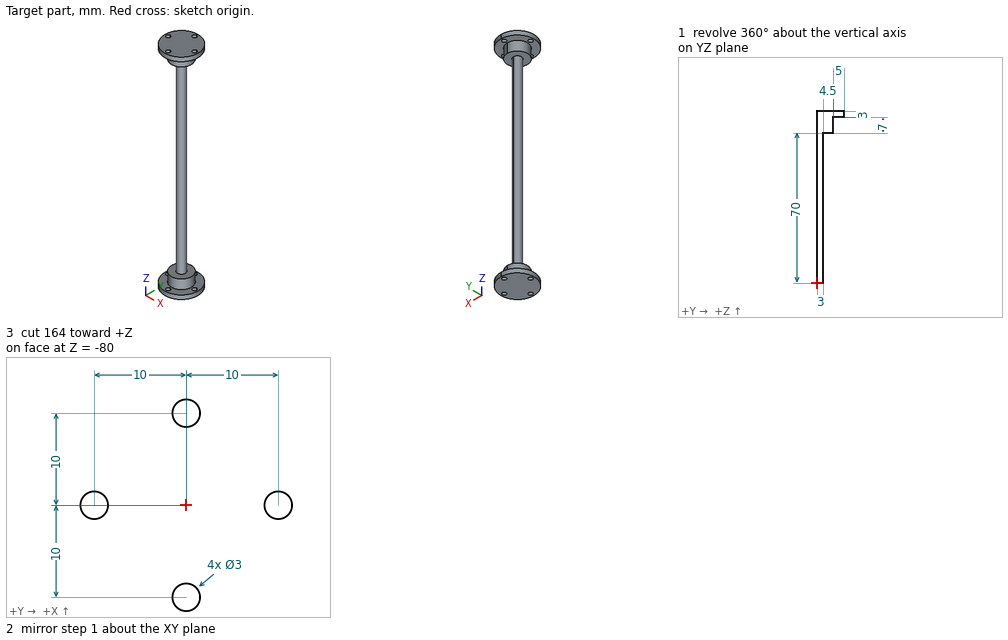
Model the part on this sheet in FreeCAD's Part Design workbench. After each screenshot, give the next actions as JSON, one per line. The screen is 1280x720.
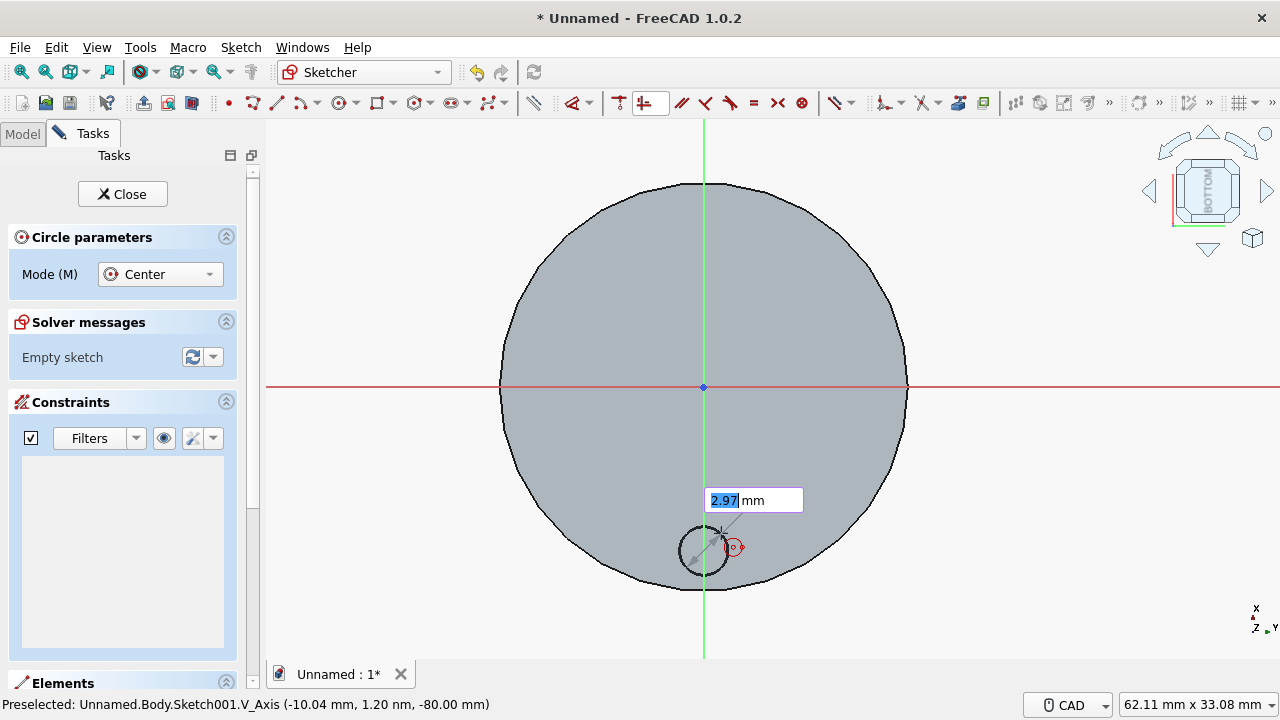
{"action": "type", "text": "3"}
{"action": "key", "text": "Return"}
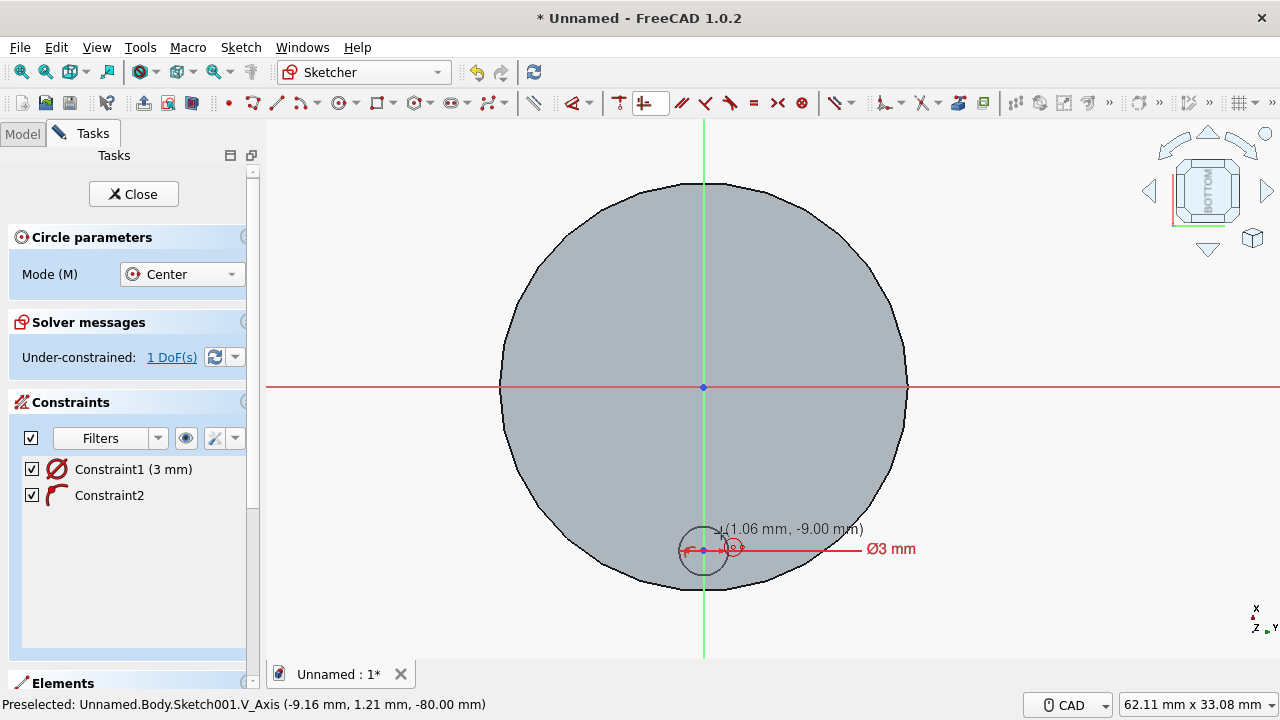
{"action": "left_click", "coordinate": [541, 387]}
{"action": "mouse_move", "coordinate": [558, 370]}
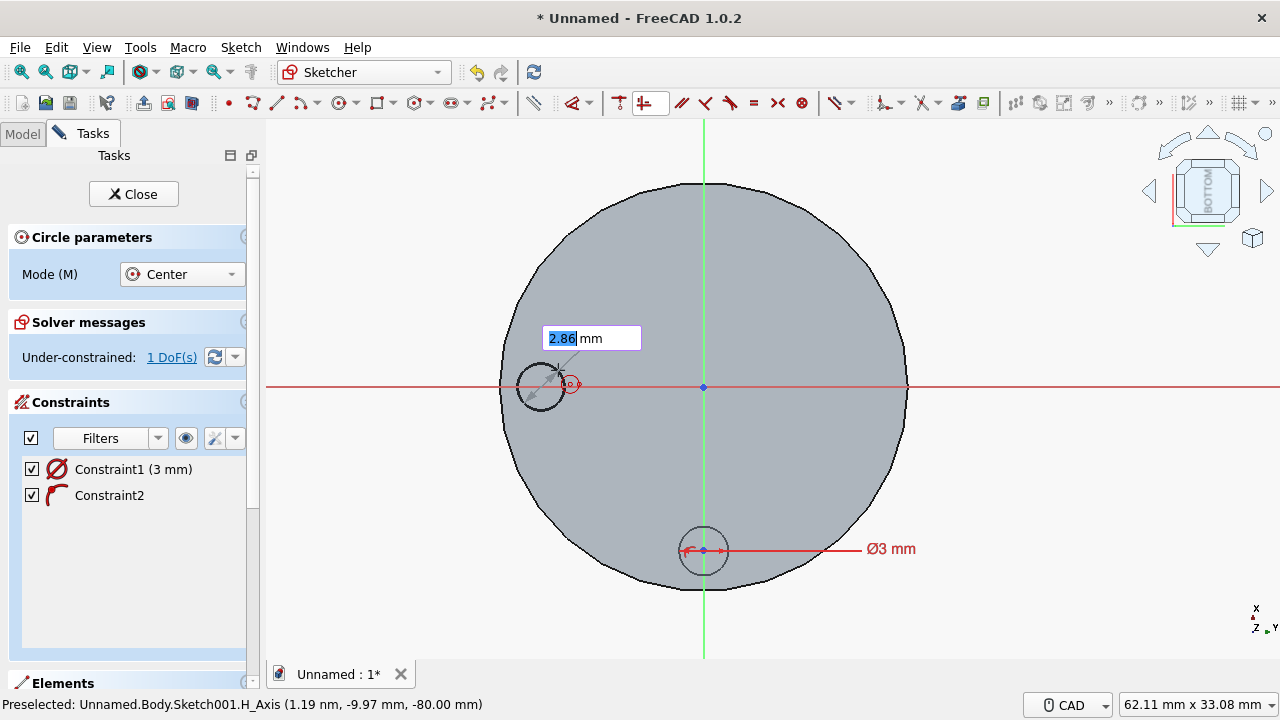
{"action": "type", "text": "3"}
{"action": "key", "text": "Return"}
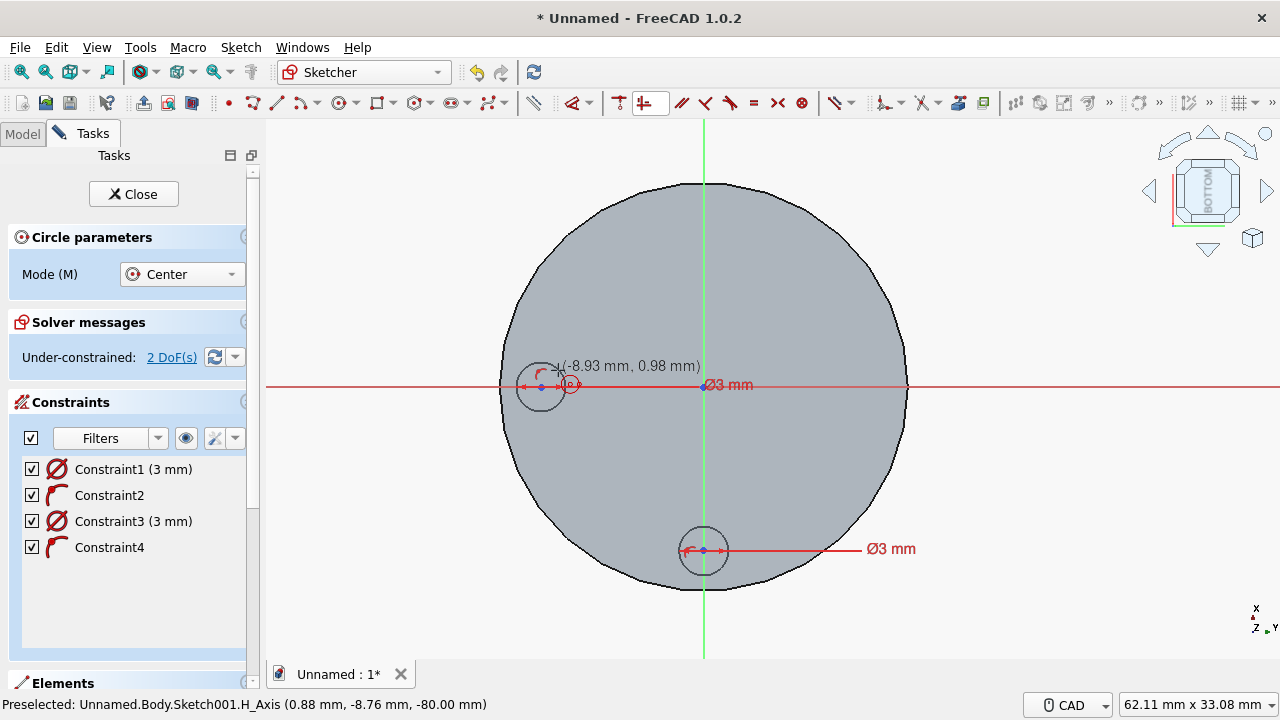
{"action": "left_click", "coordinate": [704, 224]}
{"action": "mouse_move", "coordinate": [721, 206]}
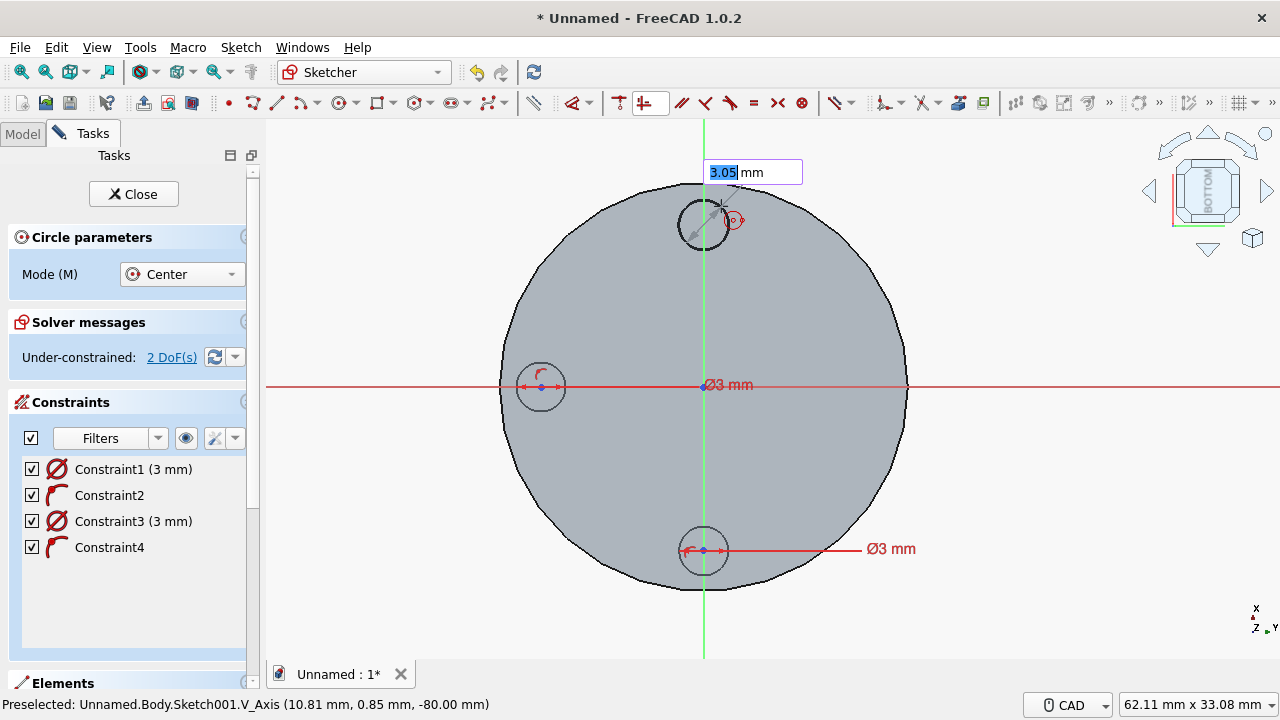
{"action": "type", "text": "3"}
{"action": "key", "text": "Return"}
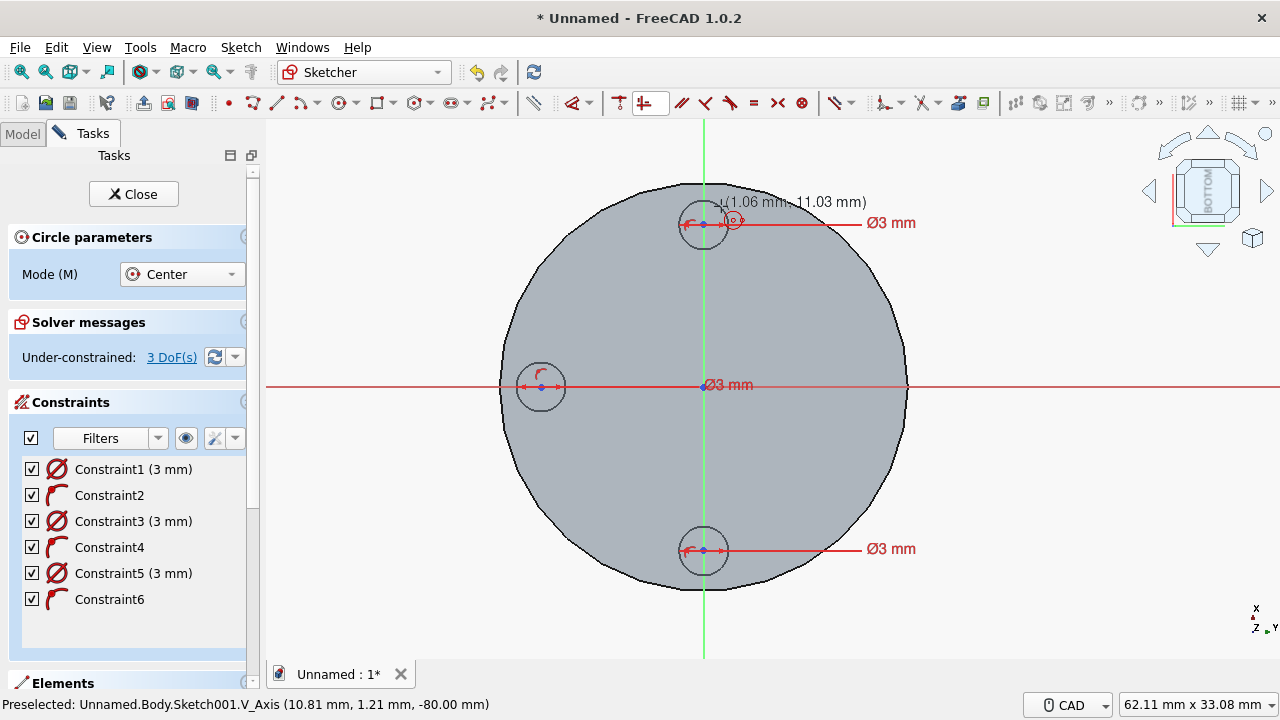
{"action": "left_click", "coordinate": [867, 387]}
{"action": "mouse_move", "coordinate": [884, 370]}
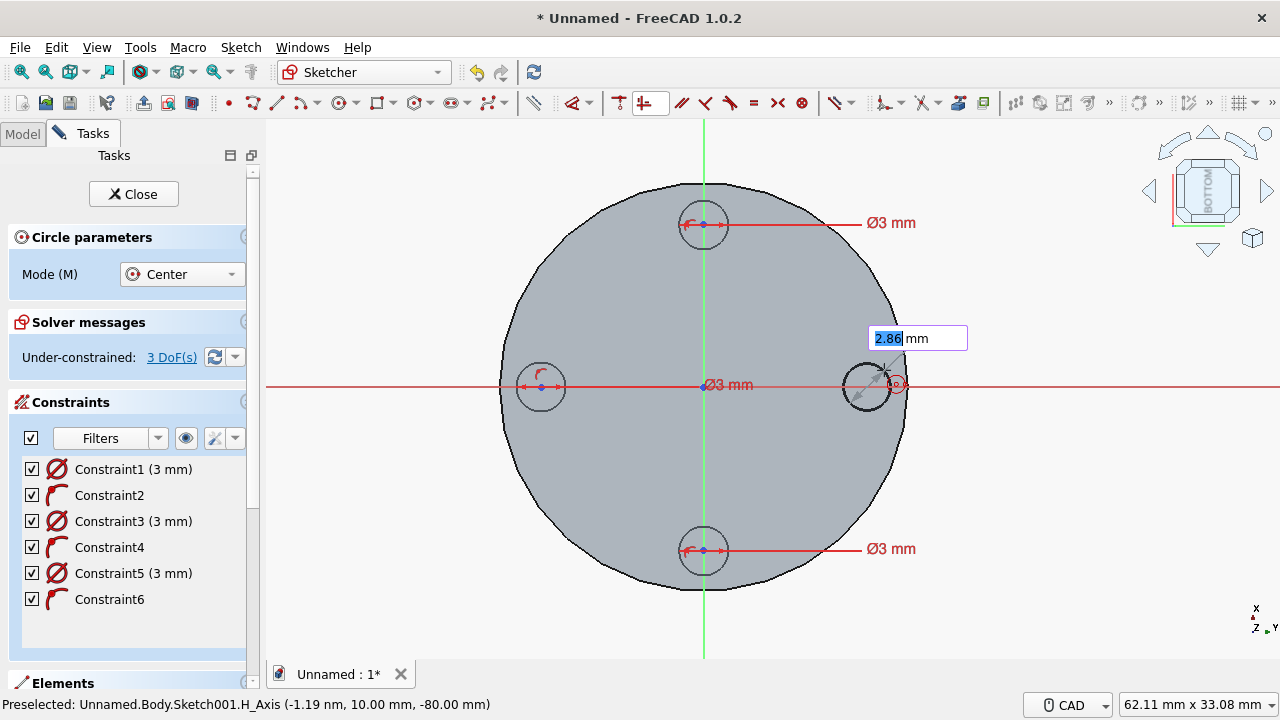
{"action": "type", "text": "3"}
{"action": "key", "text": "Return"}
{"action": "key", "text": "Escape"}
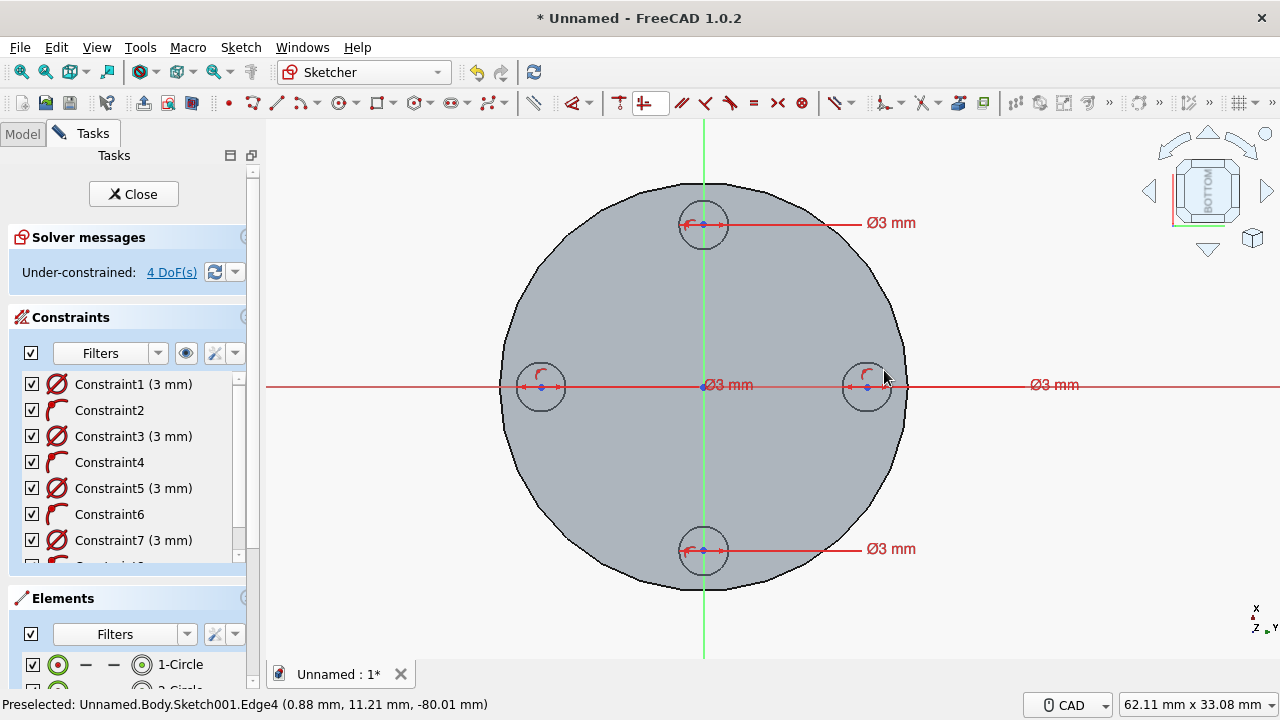
{"action": "left_click", "coordinate": [572, 104]}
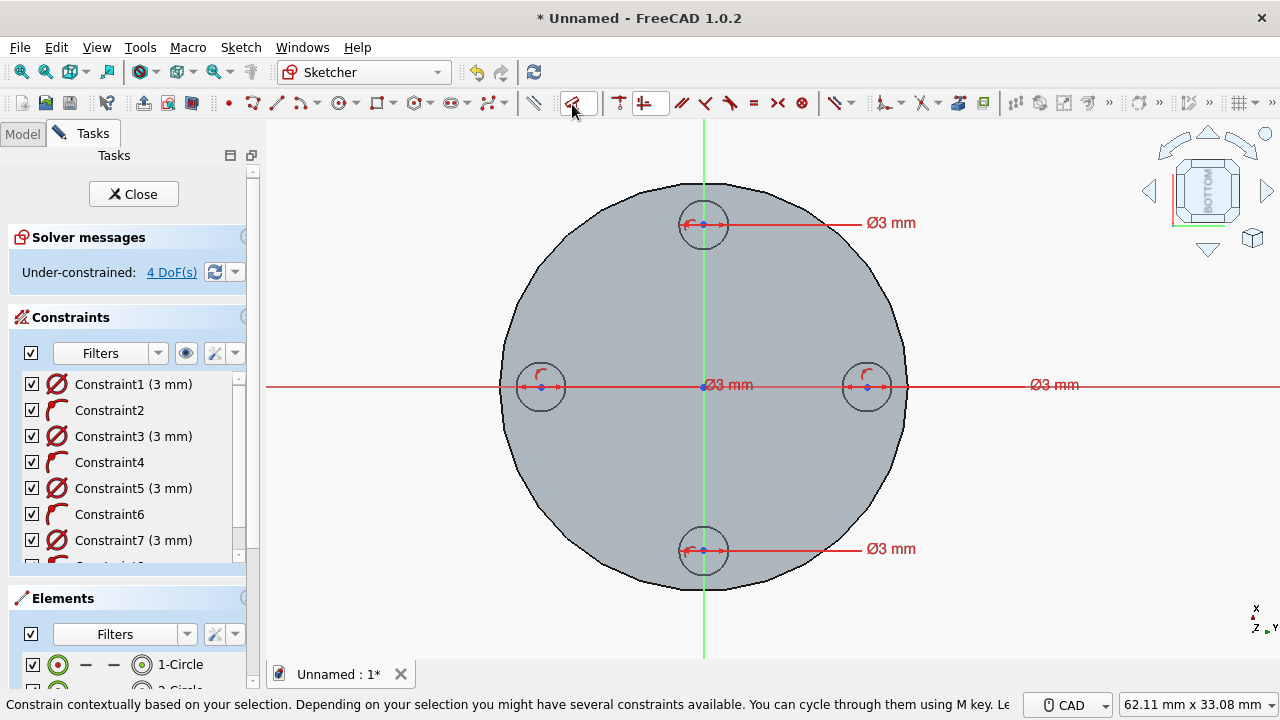
{"action": "left_click", "coordinate": [704, 551]}
{"action": "left_click", "coordinate": [738, 469]}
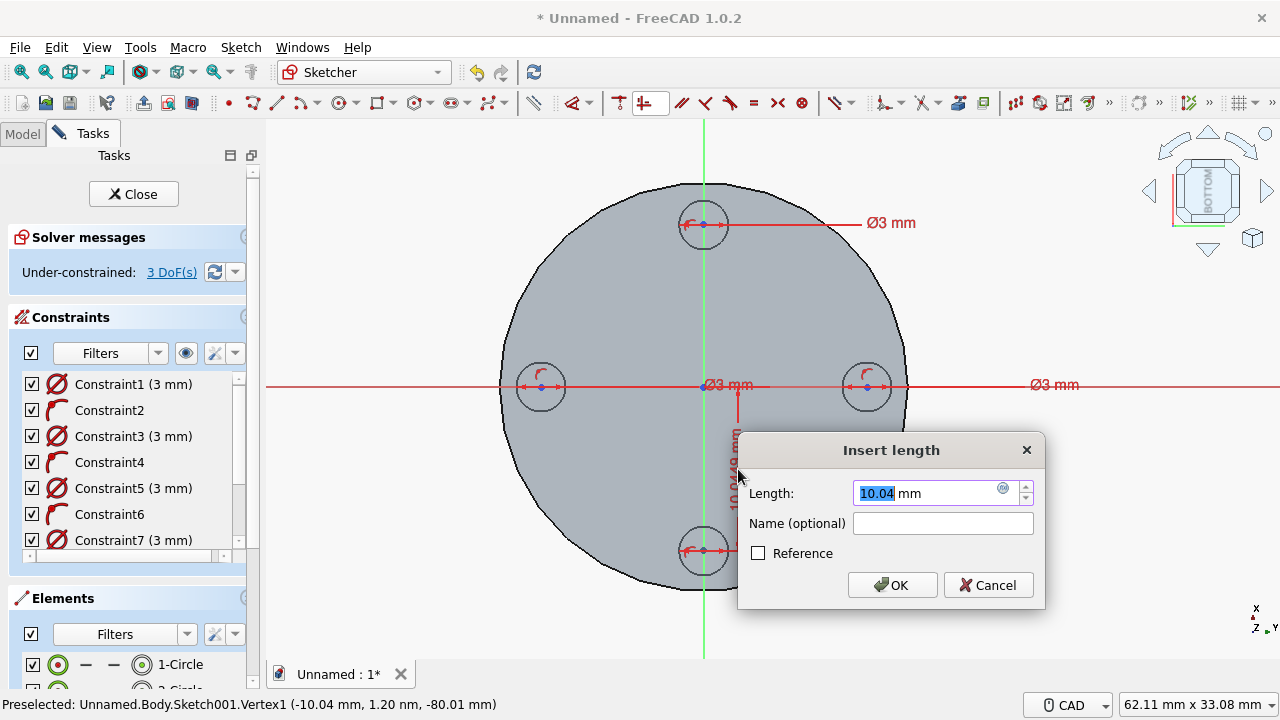
{"action": "type", "text": "10"}
{"action": "key", "text": "Return"}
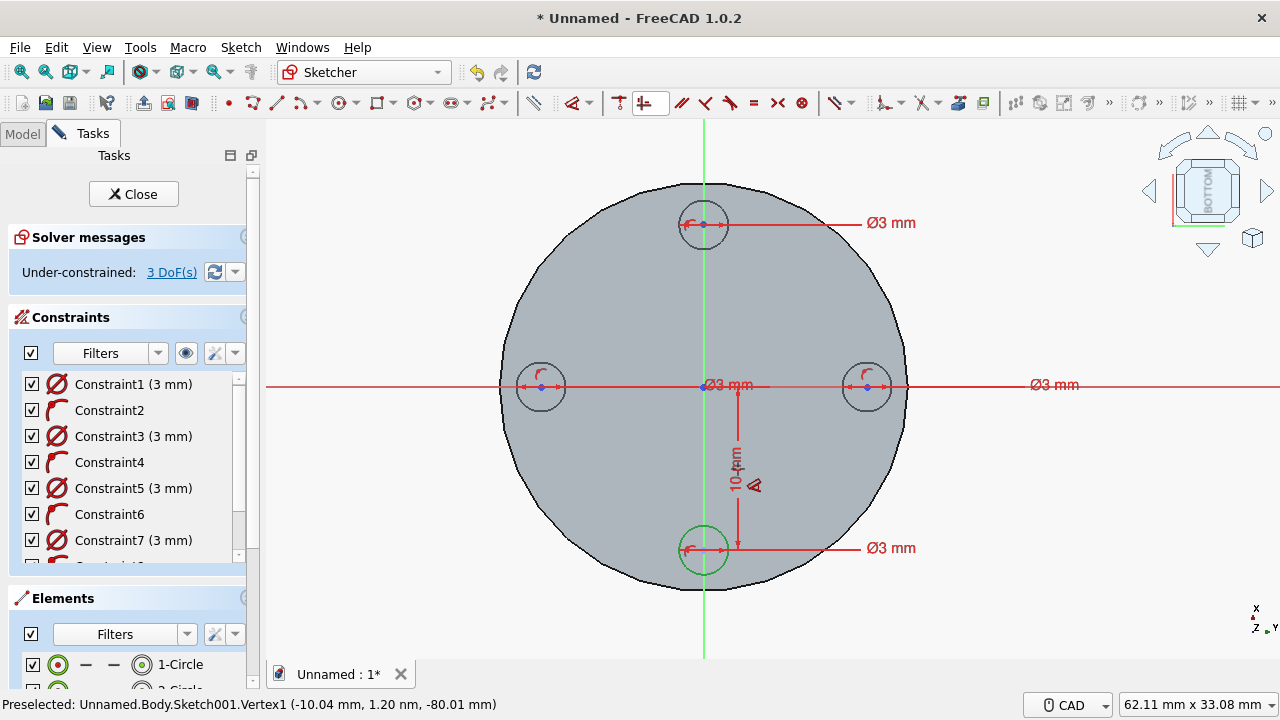
{"action": "left_click", "coordinate": [541, 387]}
{"action": "left_click", "coordinate": [622, 421]}